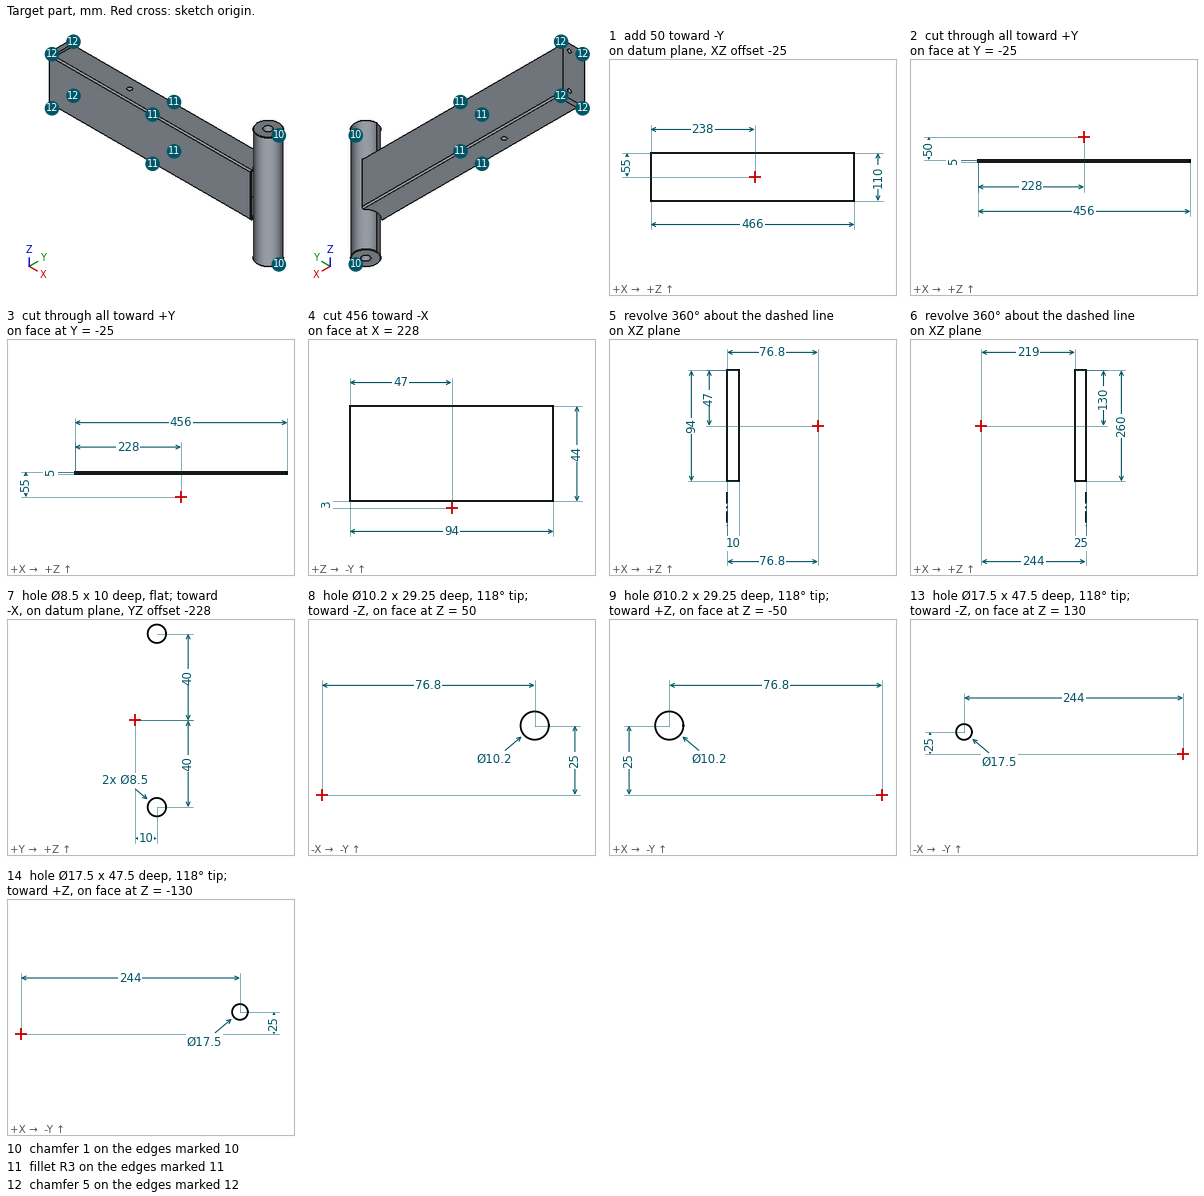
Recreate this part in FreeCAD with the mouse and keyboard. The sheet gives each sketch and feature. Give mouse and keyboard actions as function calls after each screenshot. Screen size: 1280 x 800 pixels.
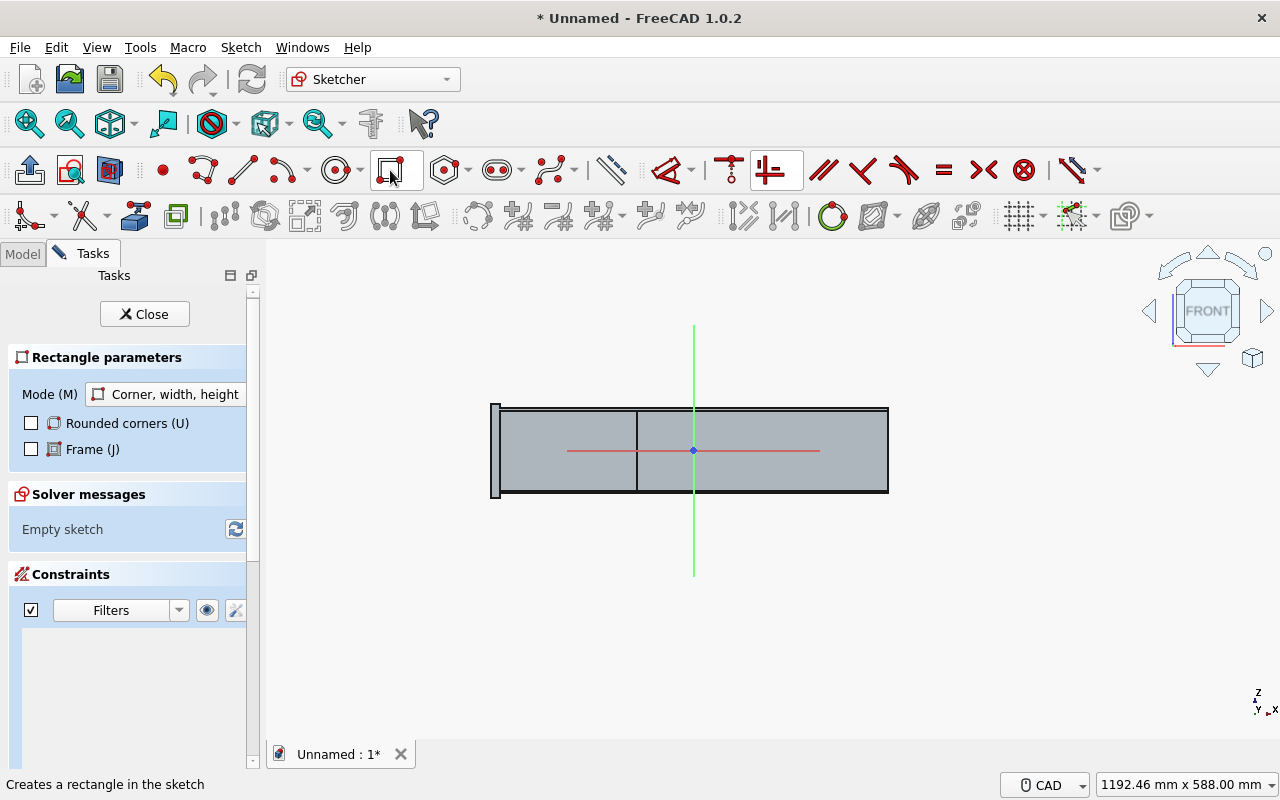
click(880, 340)
move(901, 561)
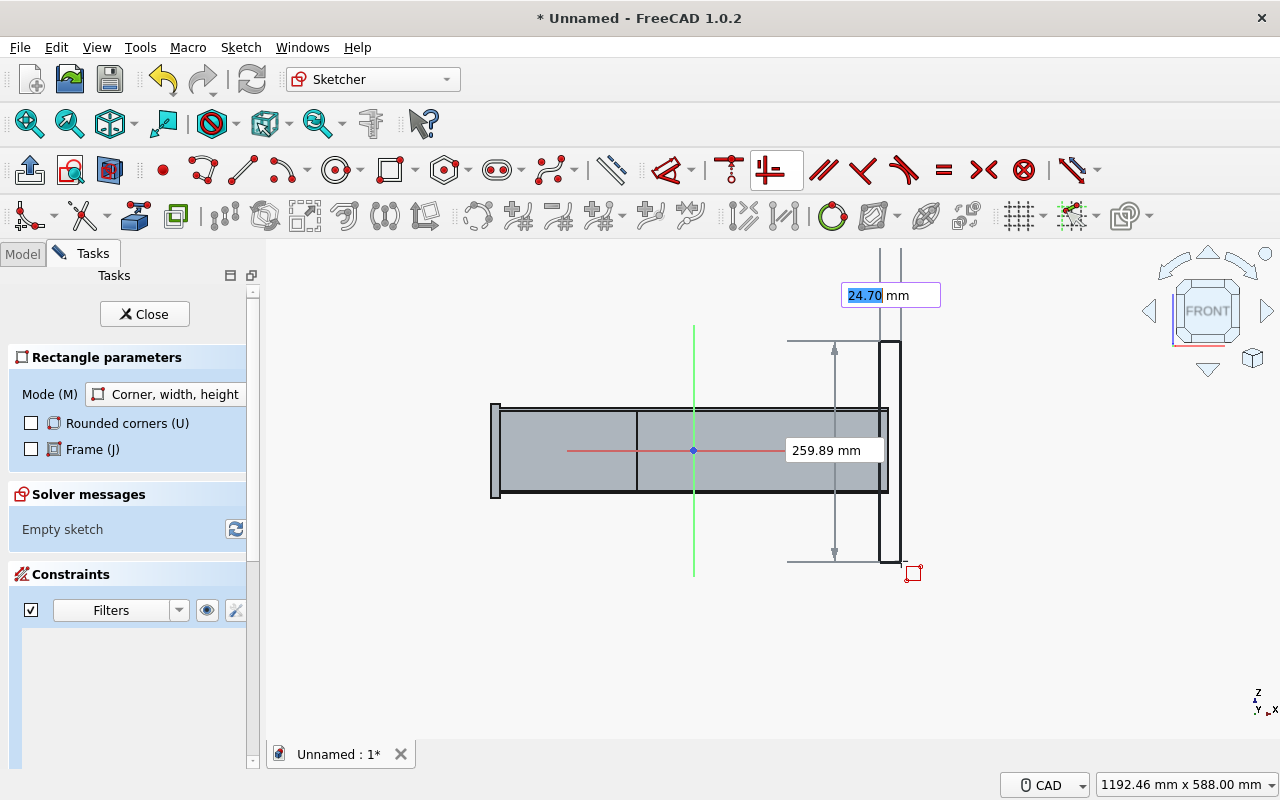
text(25)
key(Tab)
text(260)
key(Return)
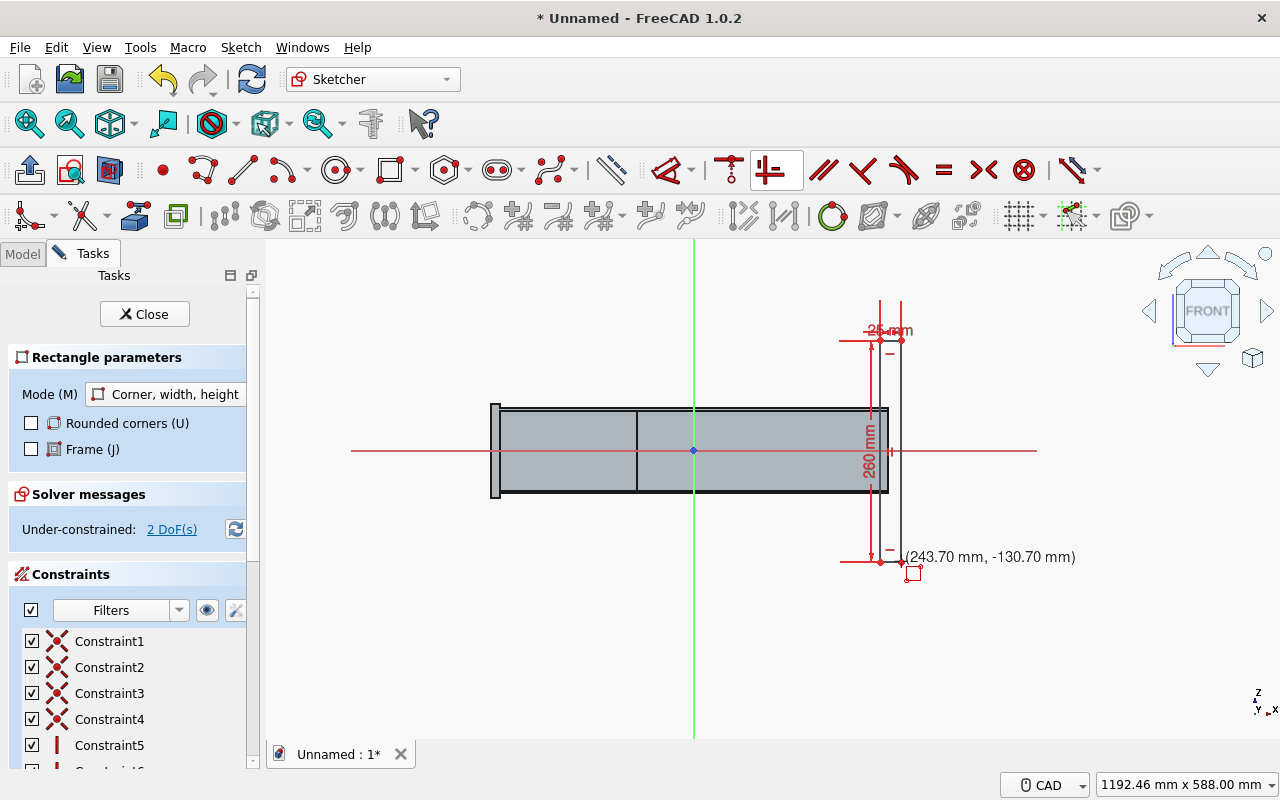
click(244, 170)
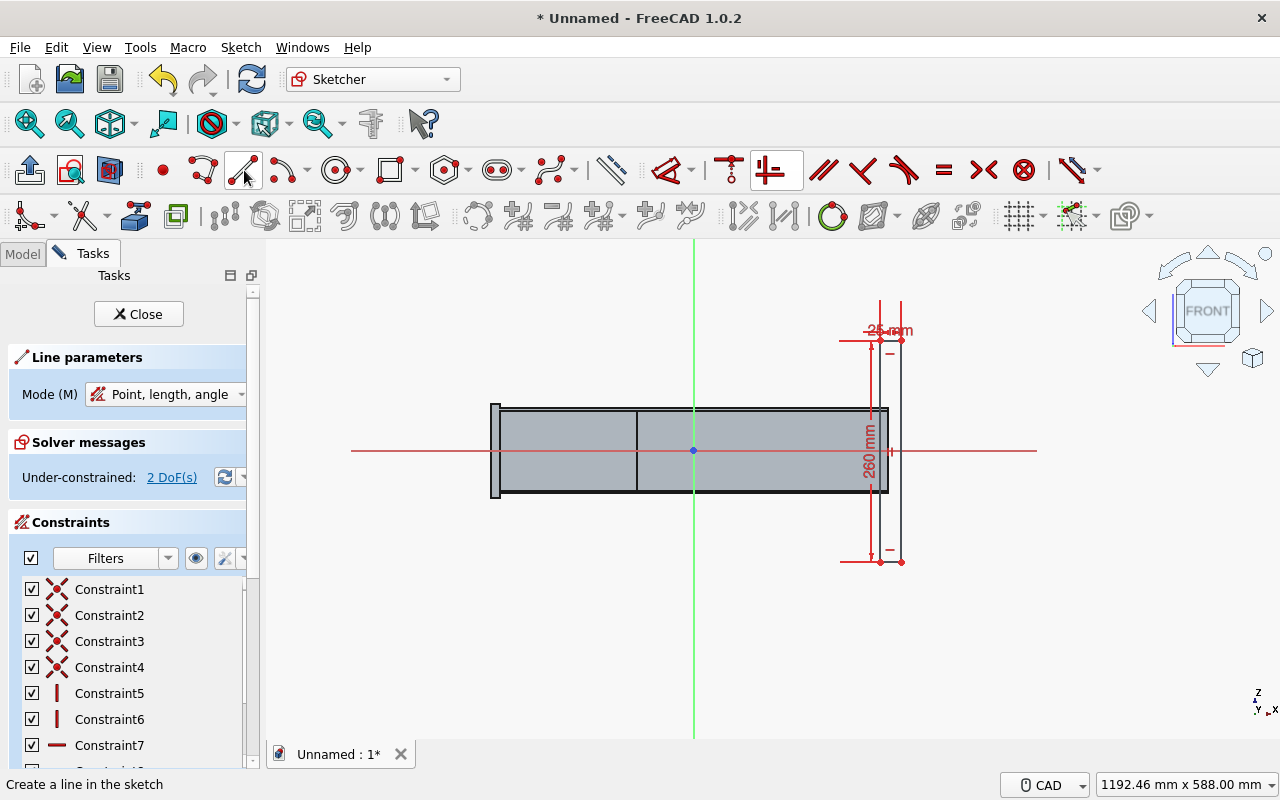
click(901, 584)
click(901, 650)
key(Escape)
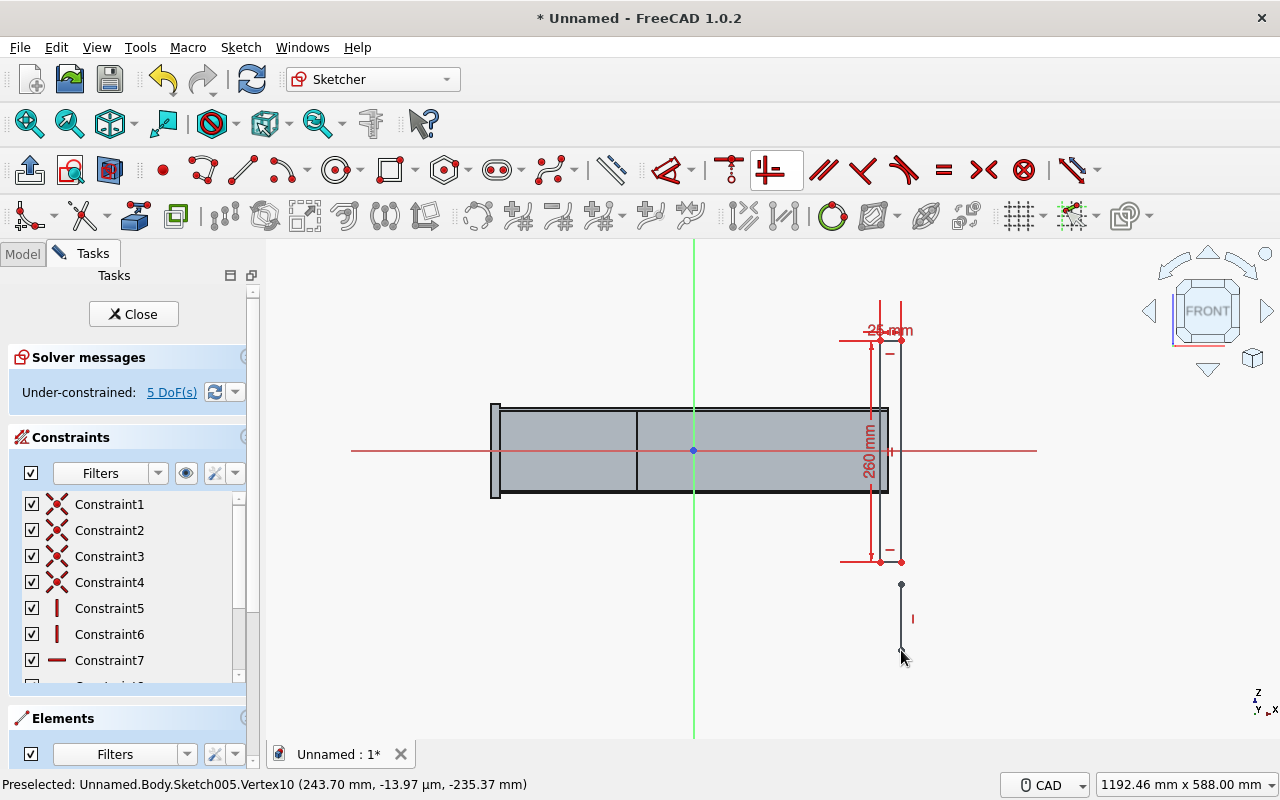
click(901, 605)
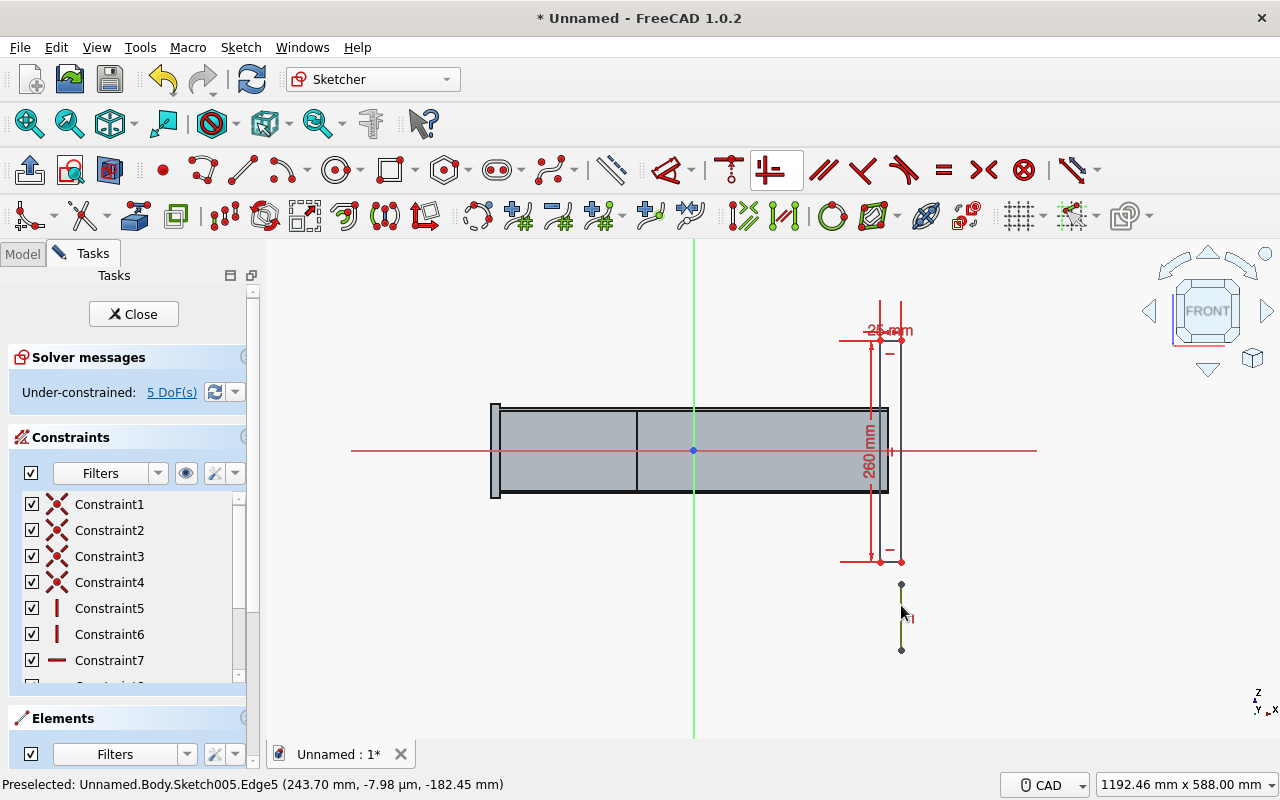
click(612, 170)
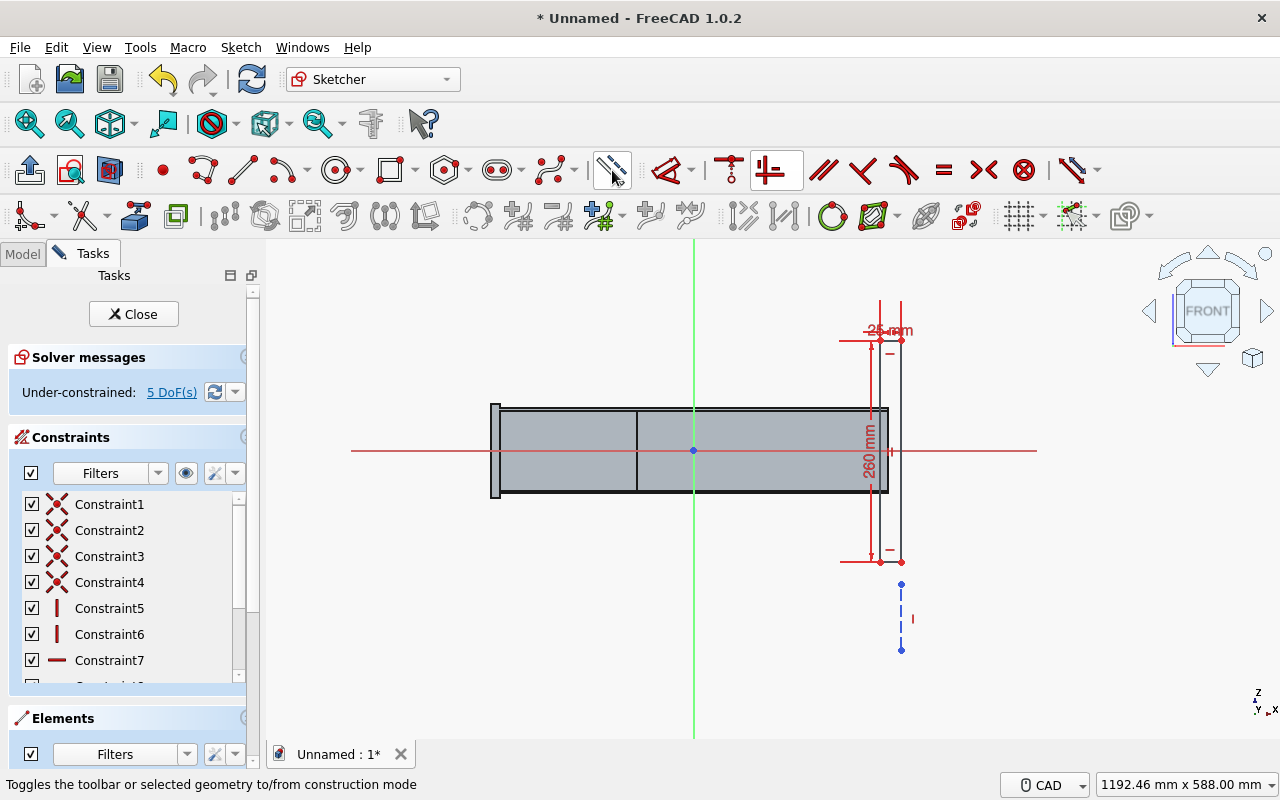
click(666, 170)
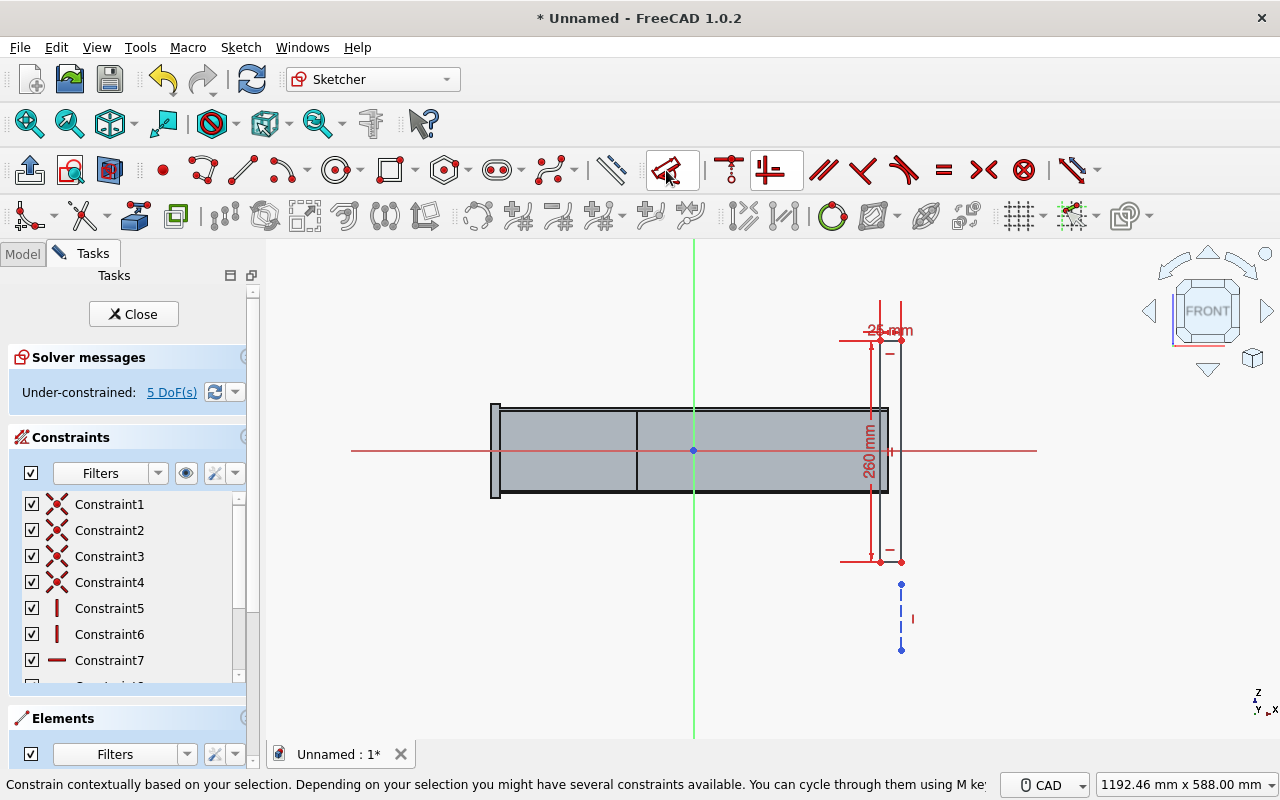
click(880, 341)
click(787, 307)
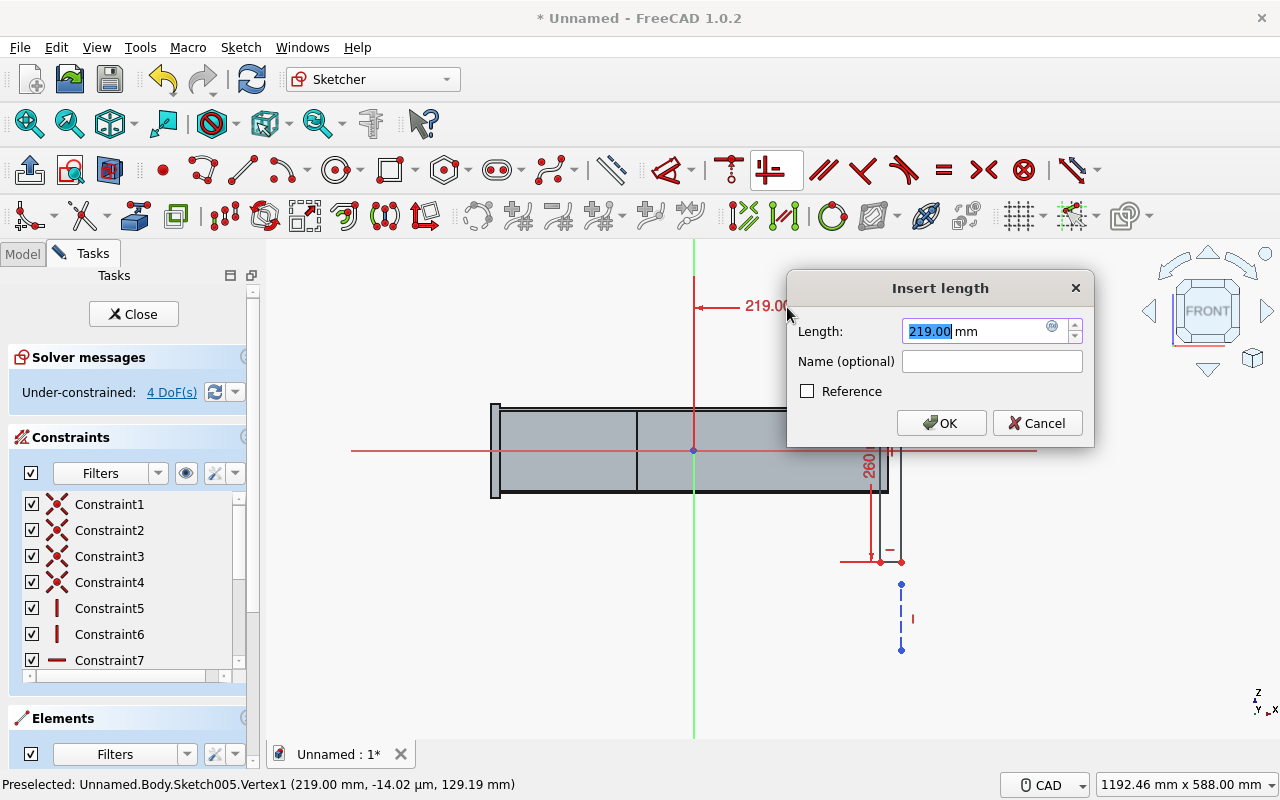
text(219)
key(Return)